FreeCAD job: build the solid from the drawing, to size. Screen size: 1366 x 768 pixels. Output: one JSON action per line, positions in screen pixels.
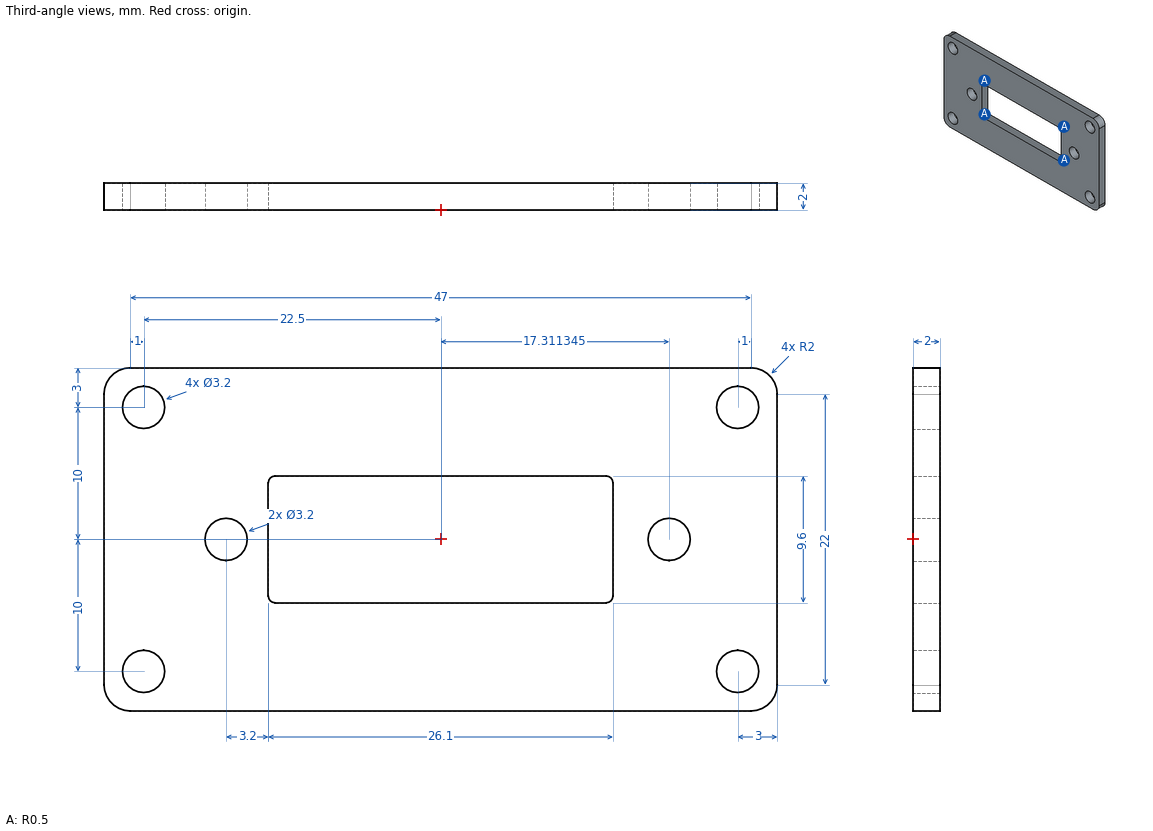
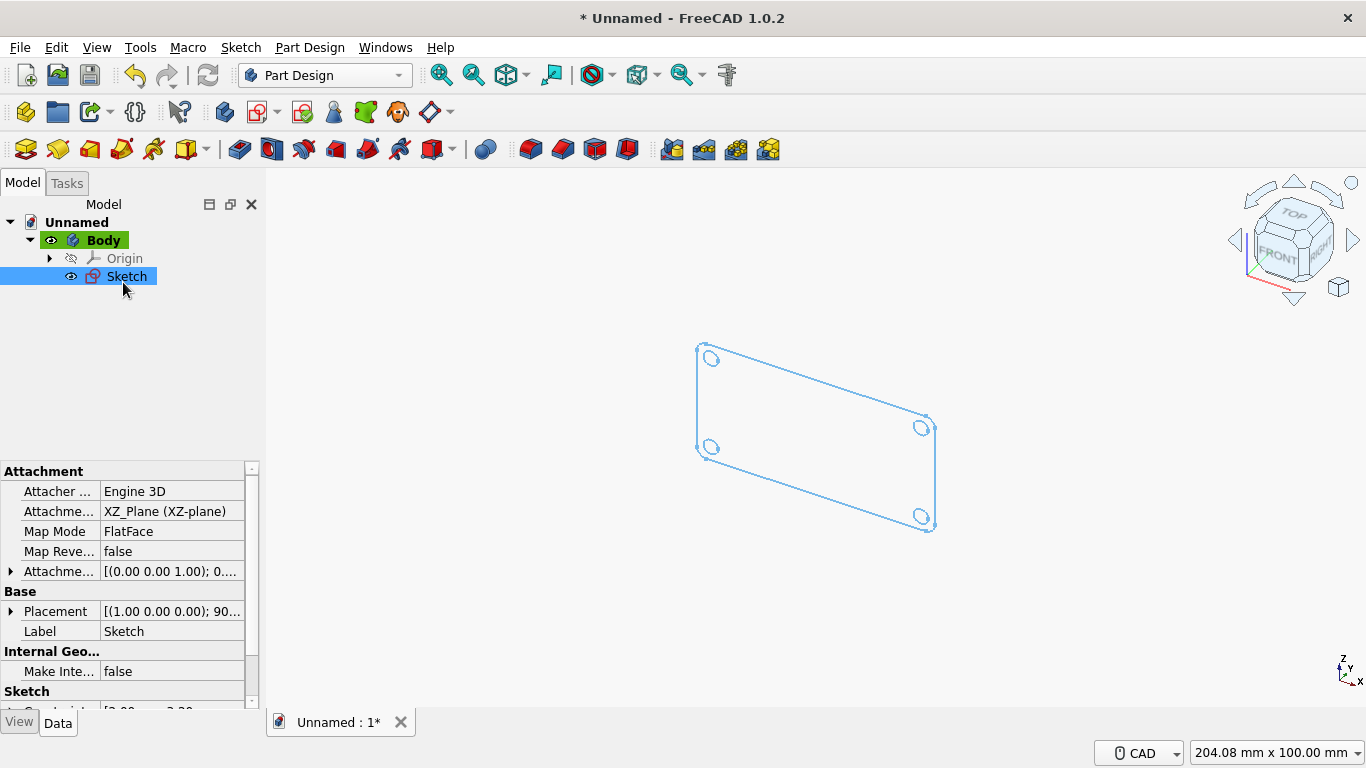
{"action": "left_click", "coordinate": [26, 150]}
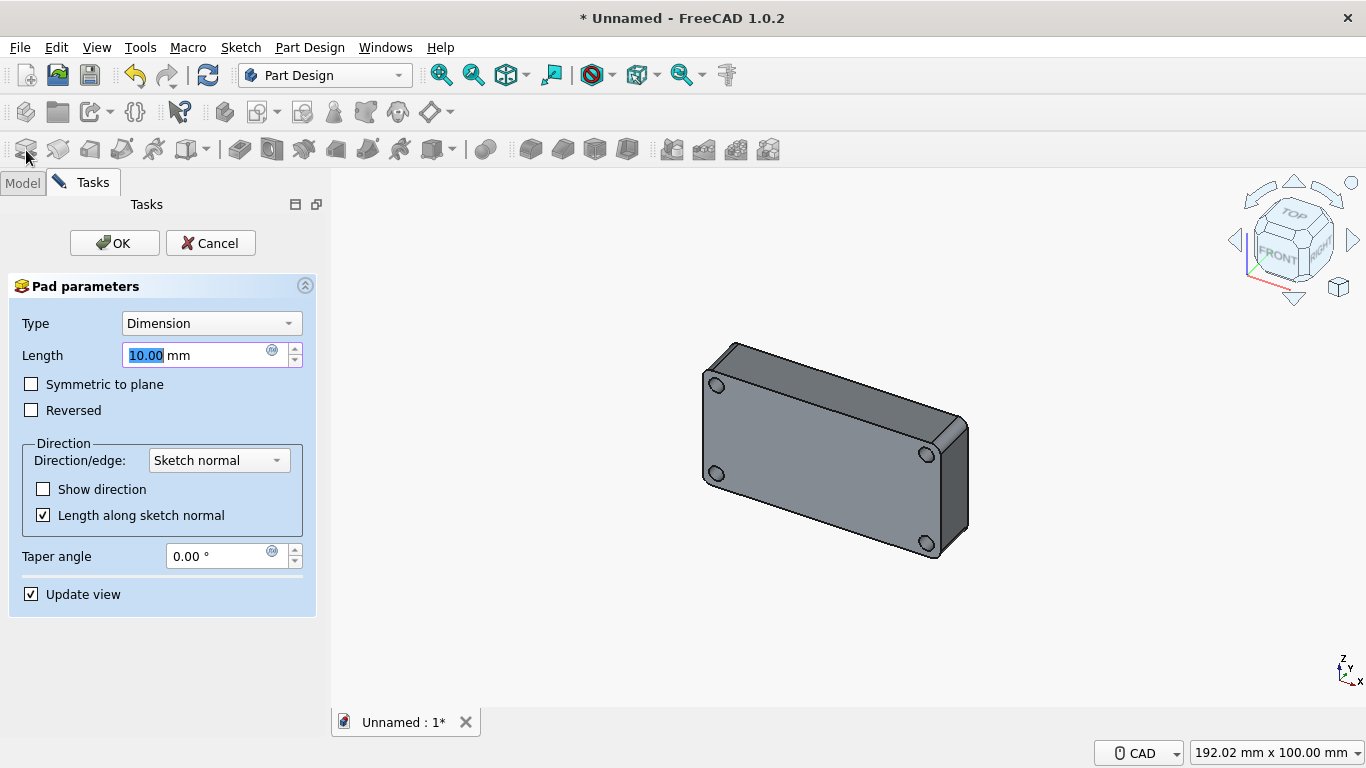
{"action": "type", "text": "2"}
{"action": "key", "text": "Tab"}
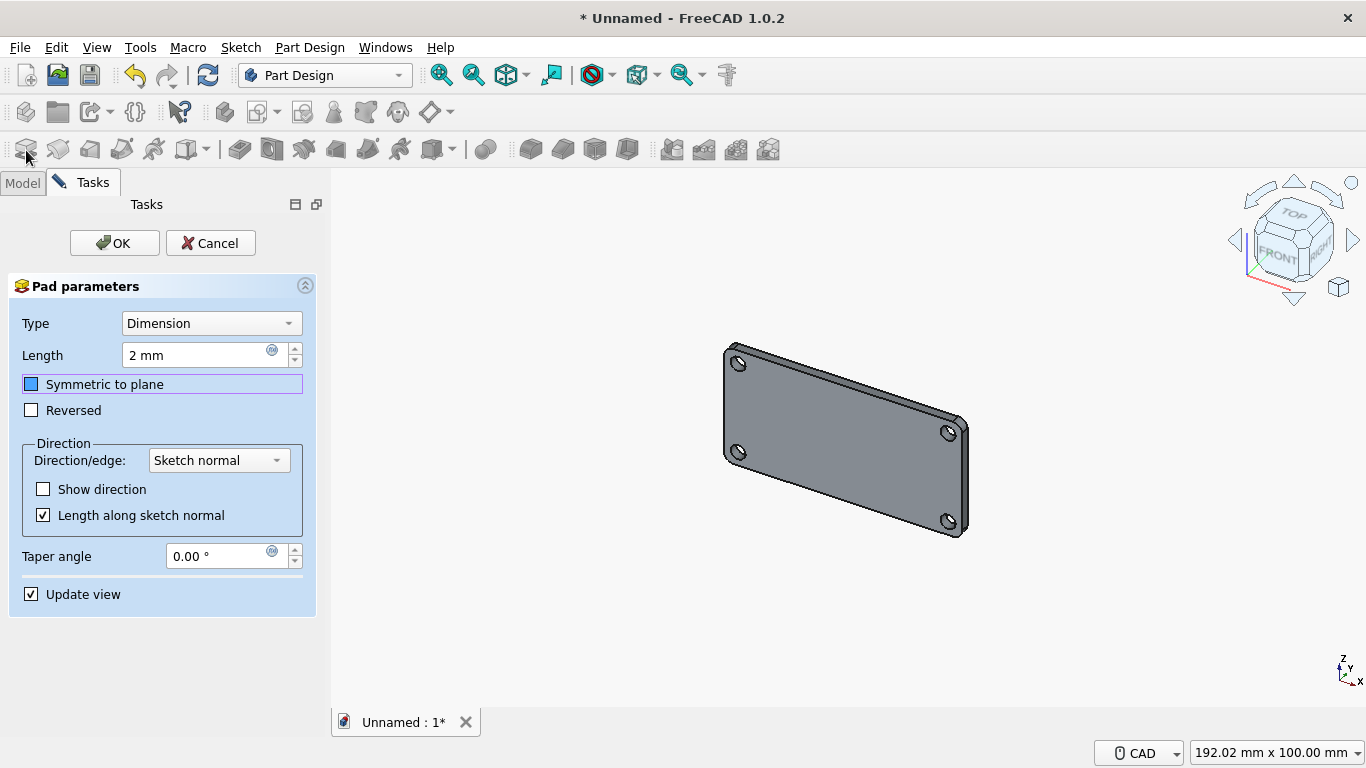
{"action": "left_click", "coordinate": [30, 410]}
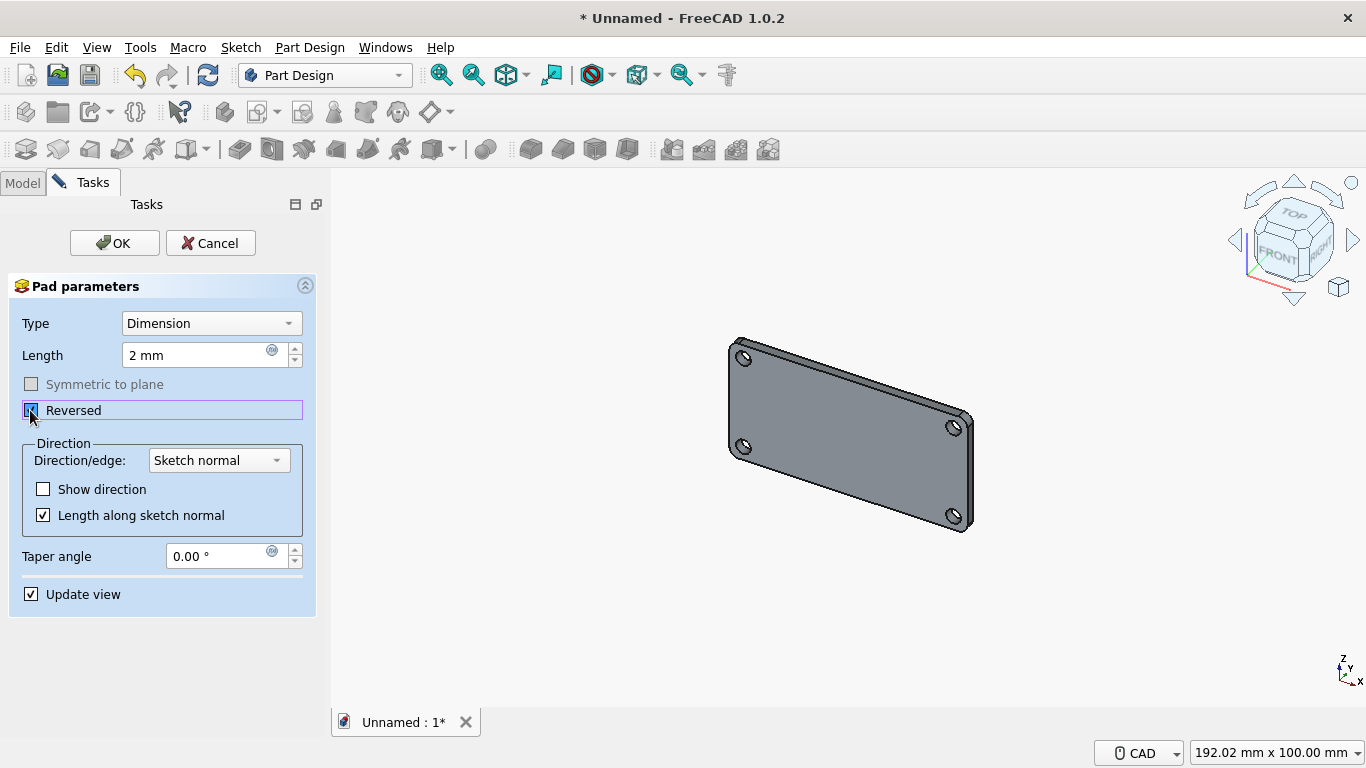
{"action": "left_click", "coordinate": [115, 243]}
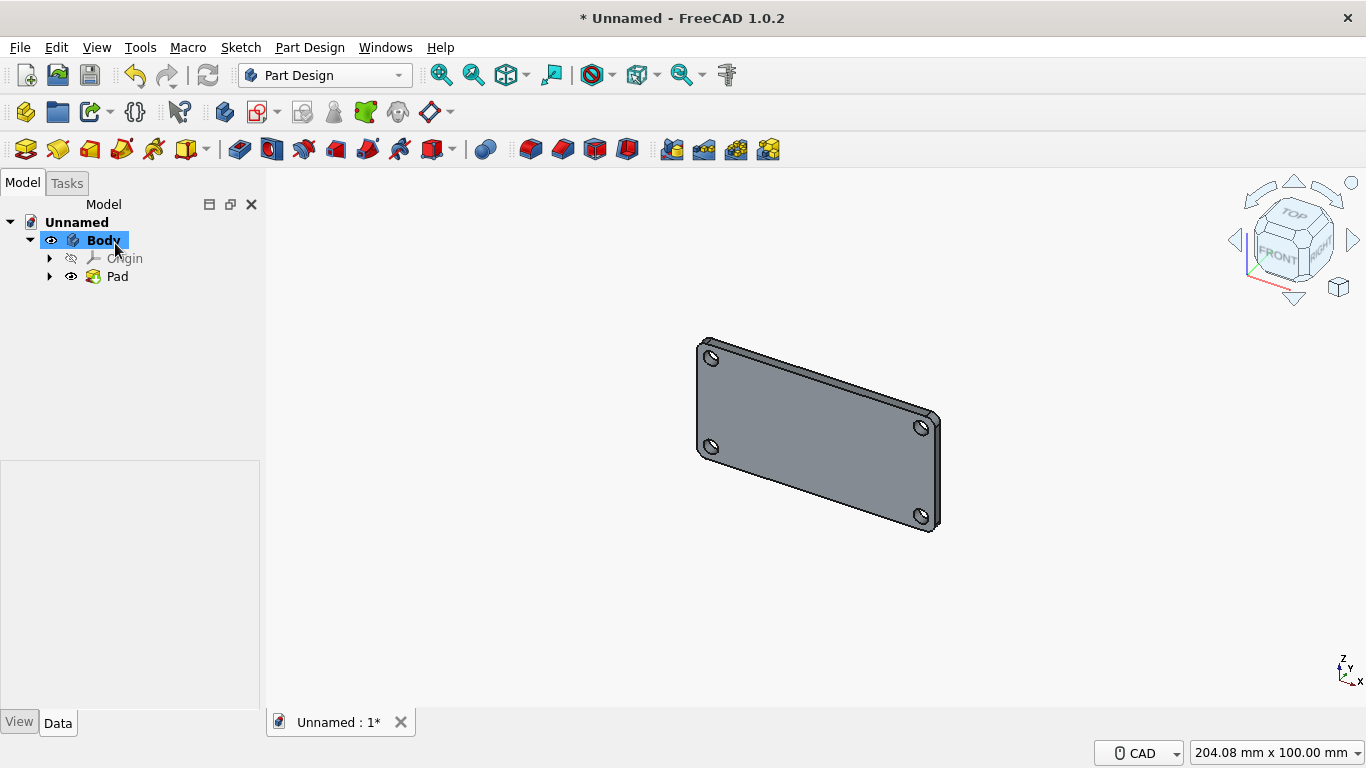
{"action": "left_click", "coordinate": [442, 76]}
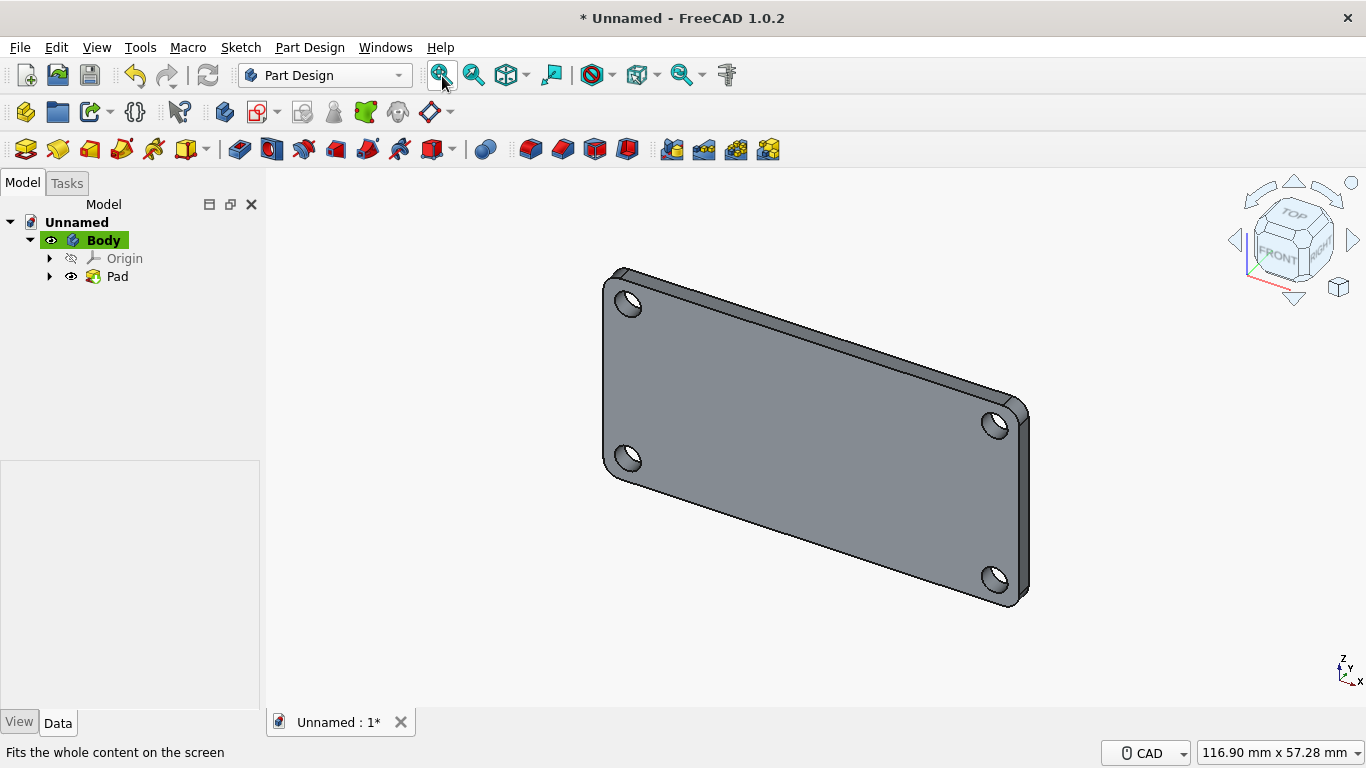
{"action": "left_click", "coordinate": [258, 112]}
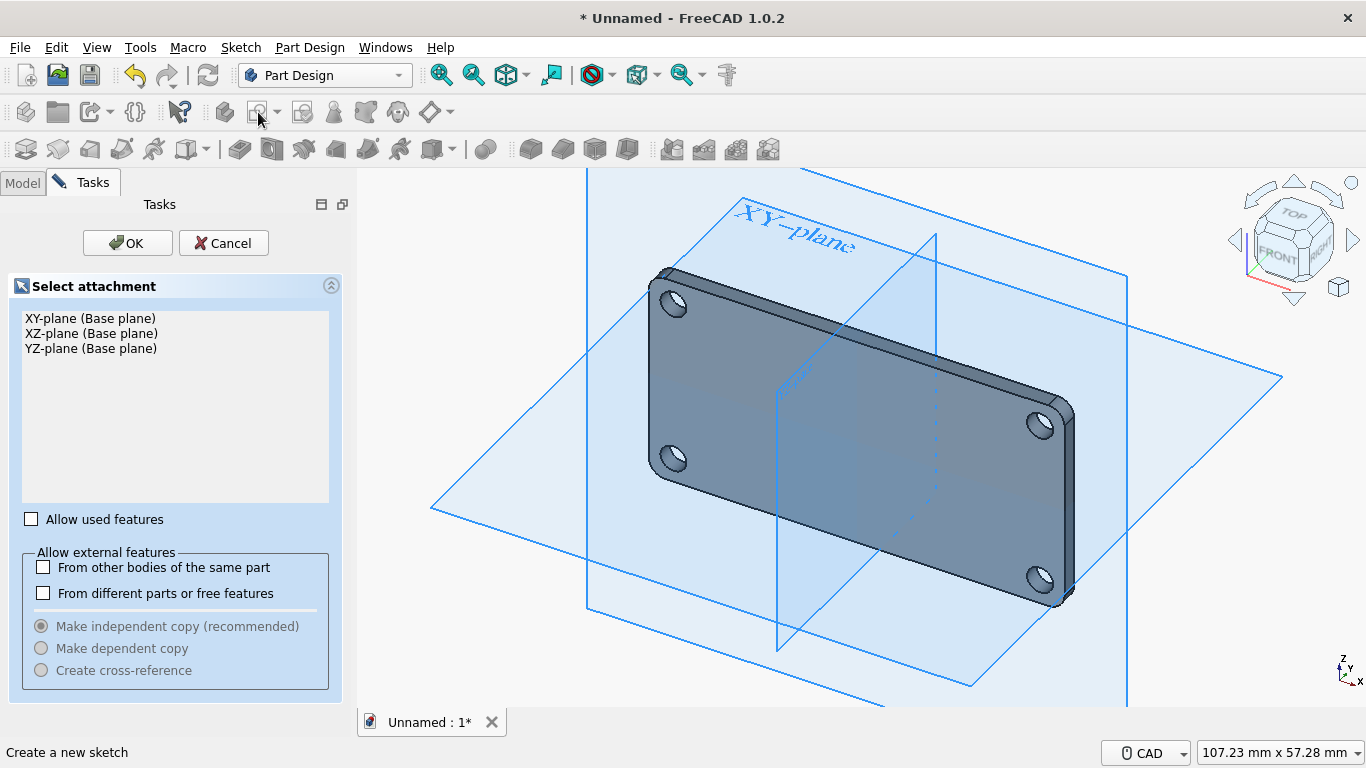
{"action": "left_click", "coordinate": [82, 334]}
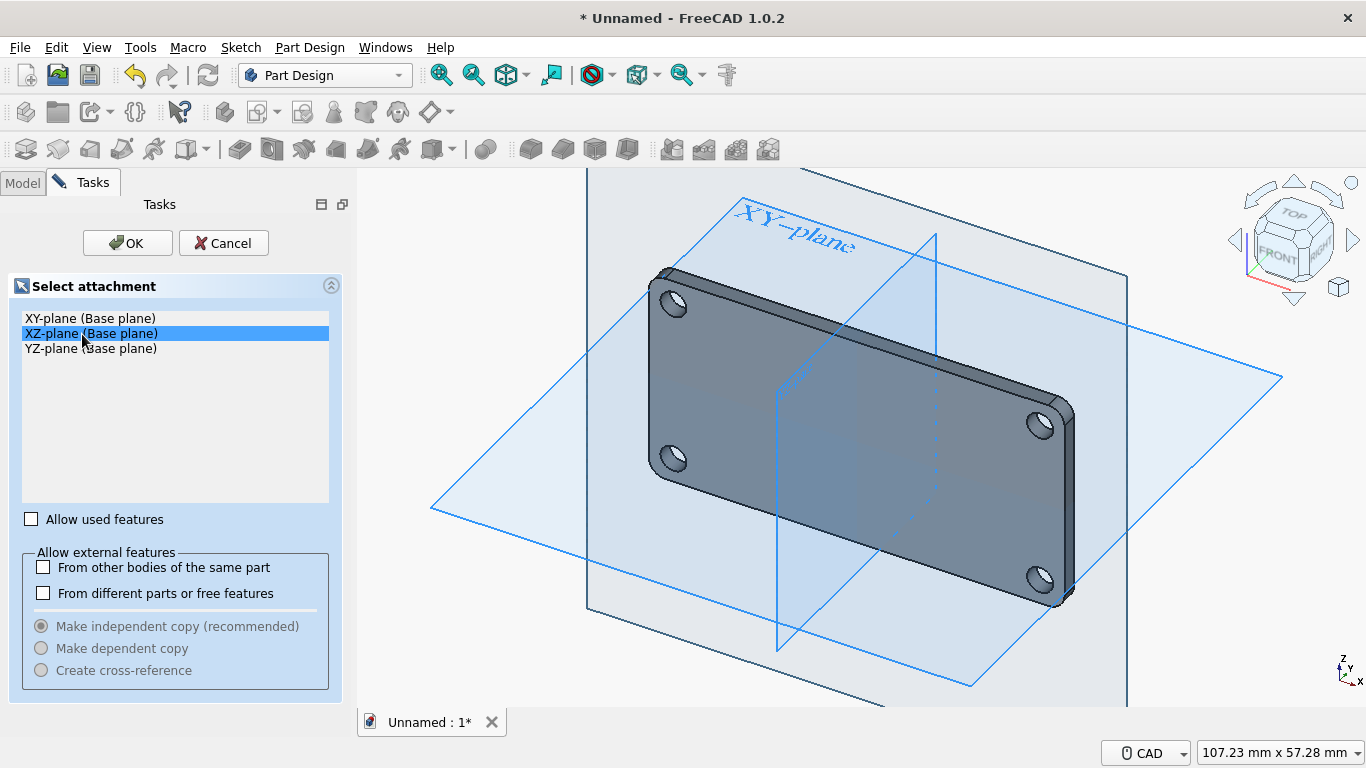
{"action": "left_click", "coordinate": [128, 243]}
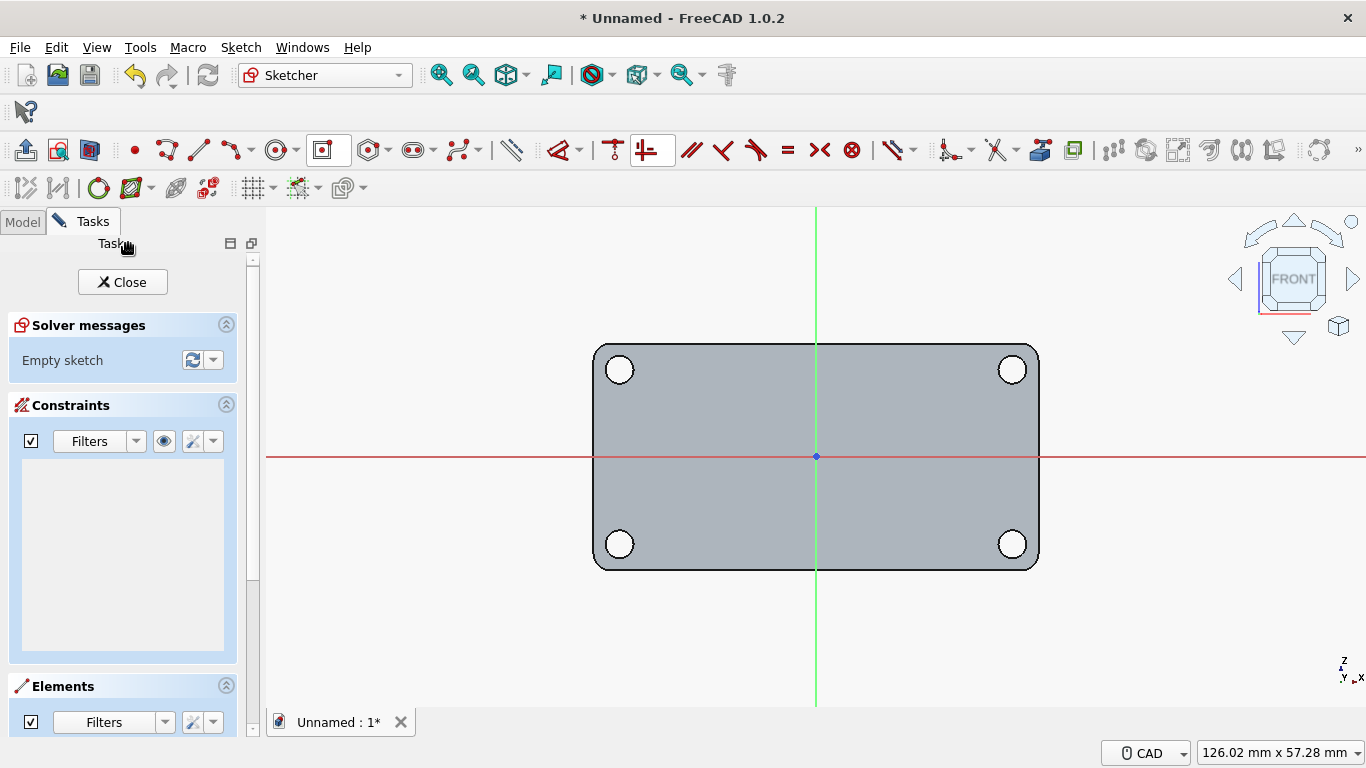
{"action": "scroll", "coordinate": [910, 457], "scroll_direction": "up", "scroll_amount": 3}